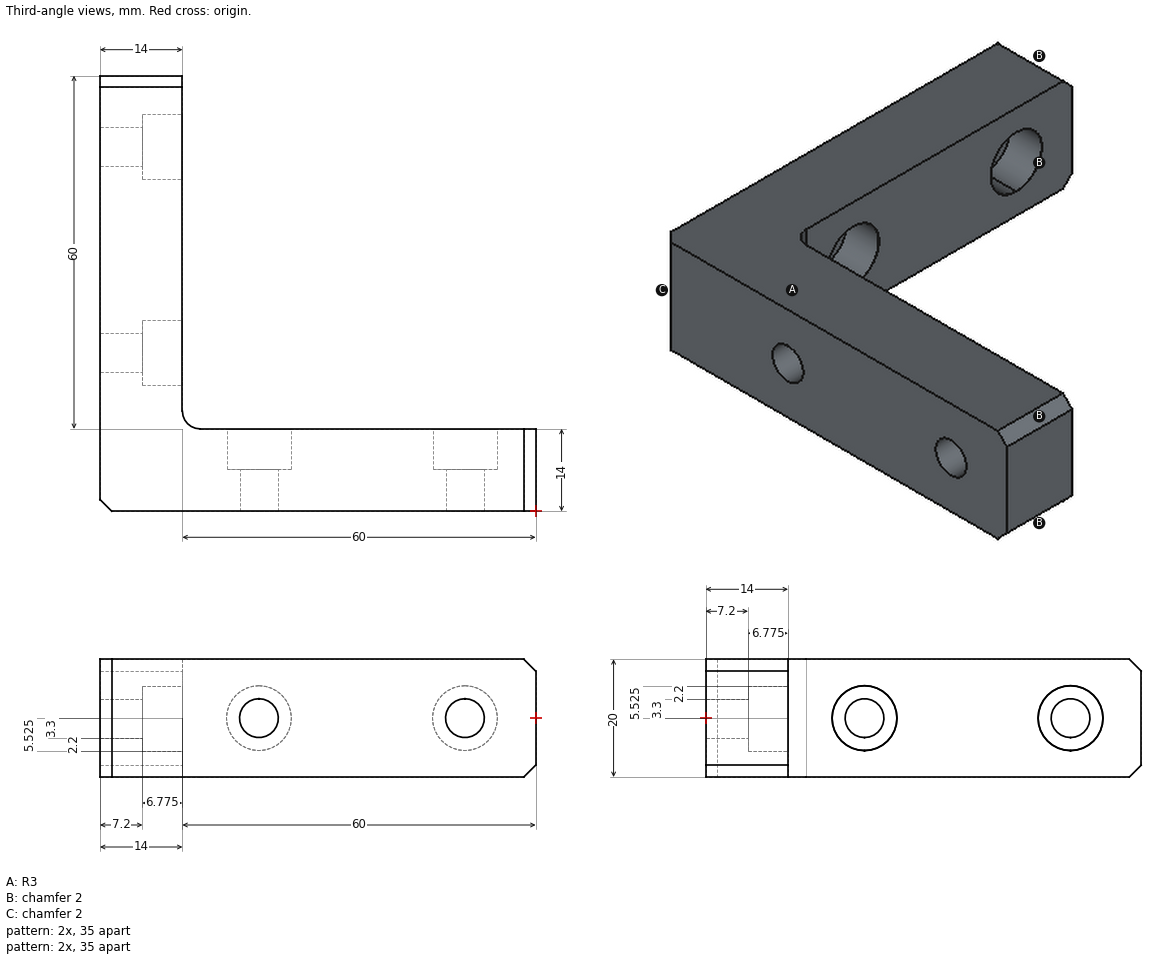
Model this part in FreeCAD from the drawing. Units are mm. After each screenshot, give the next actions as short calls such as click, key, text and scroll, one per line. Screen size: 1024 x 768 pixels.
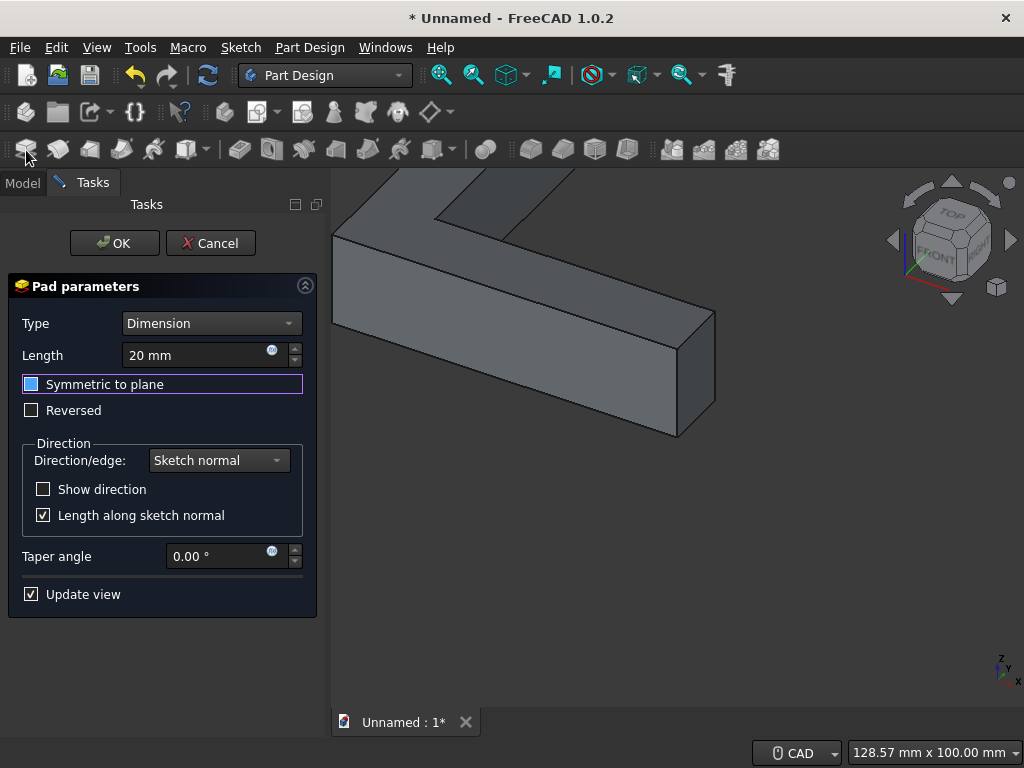
click(30, 384)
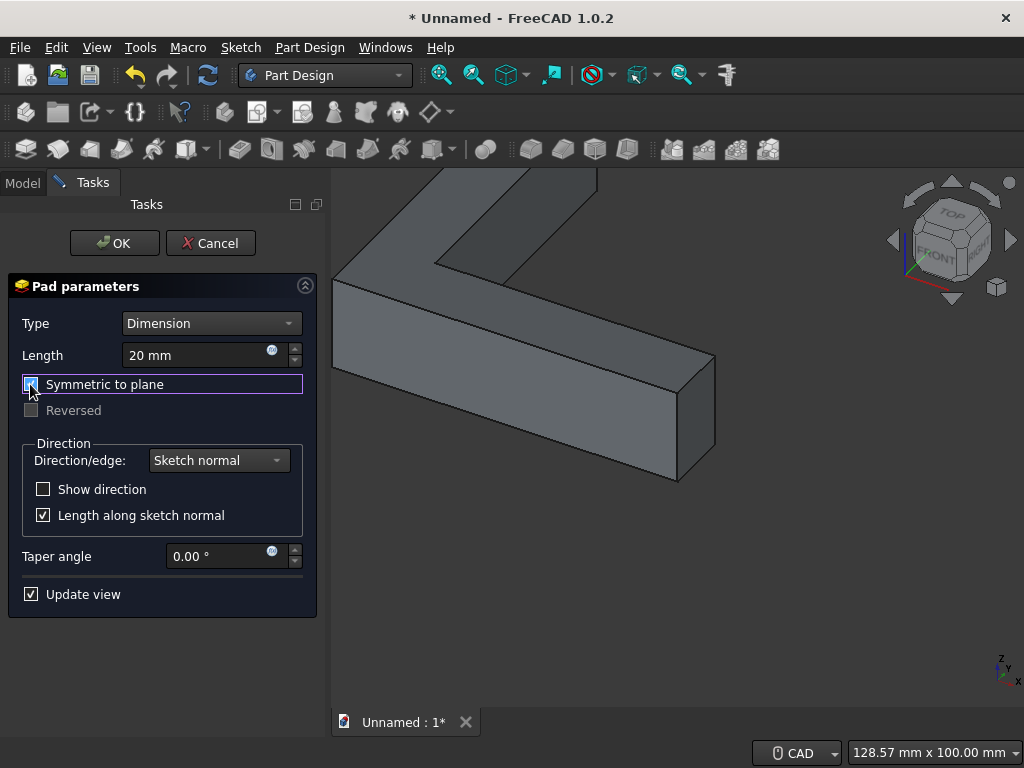
click(115, 243)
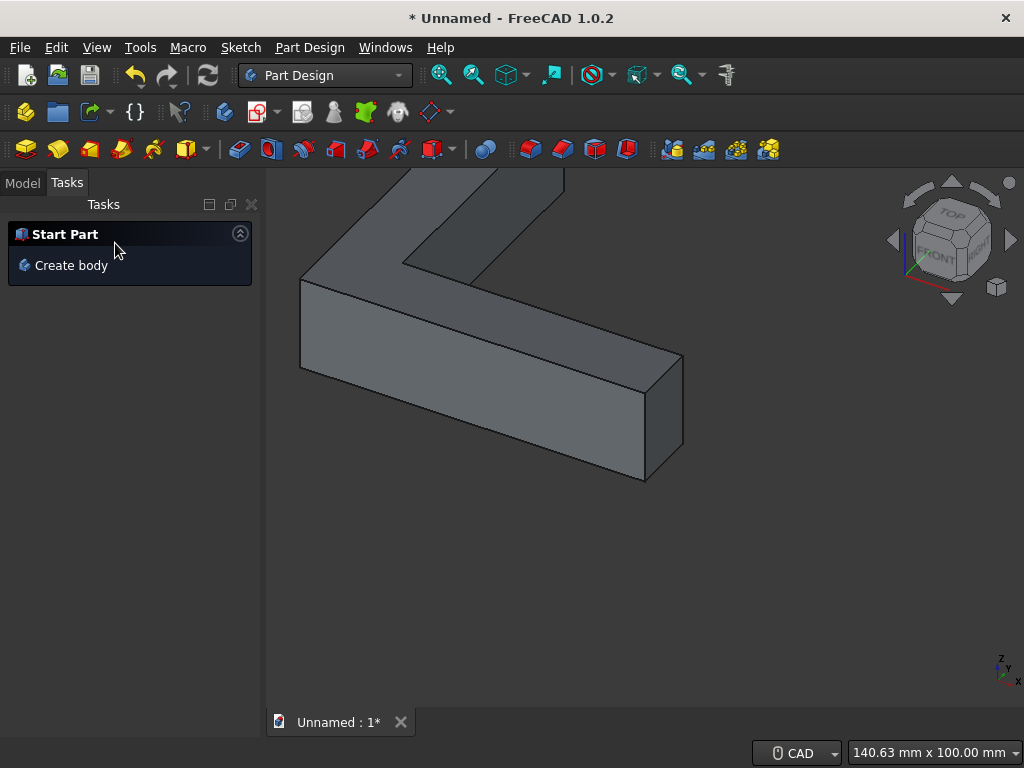
click(442, 76)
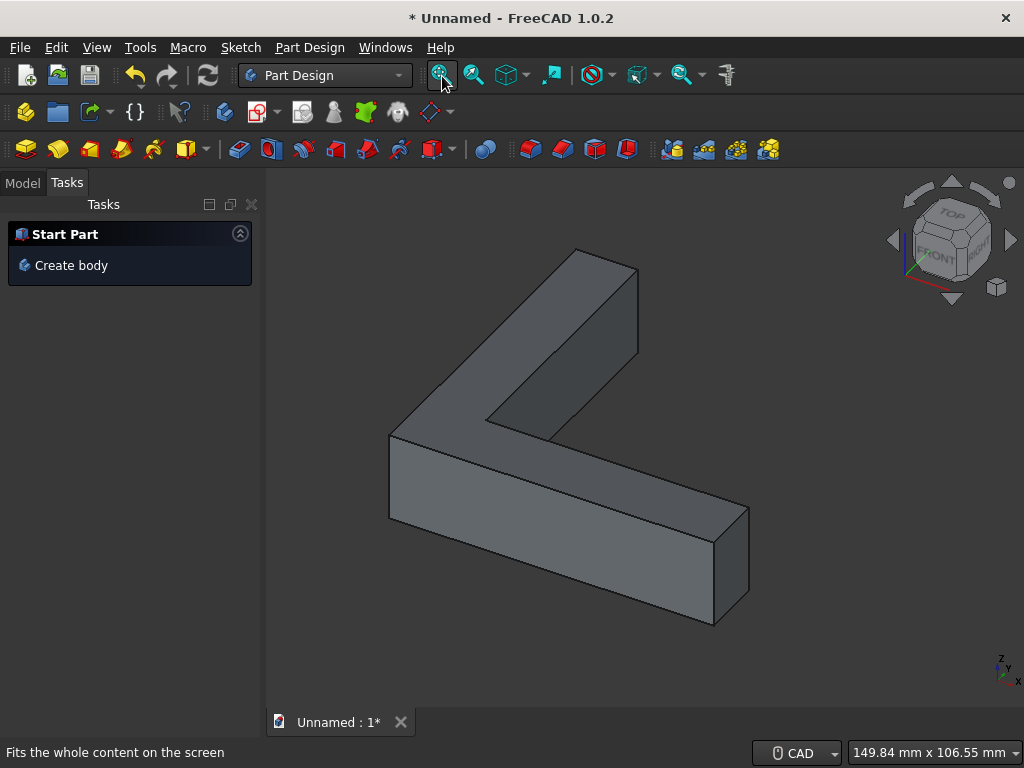
key(0)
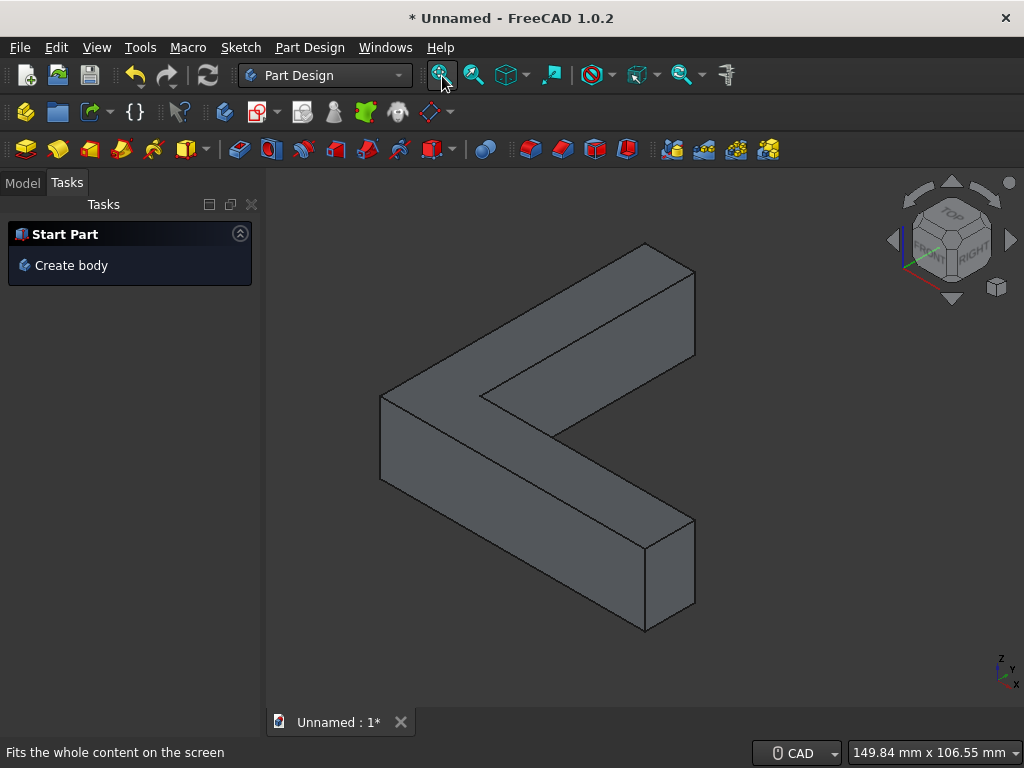
key(2)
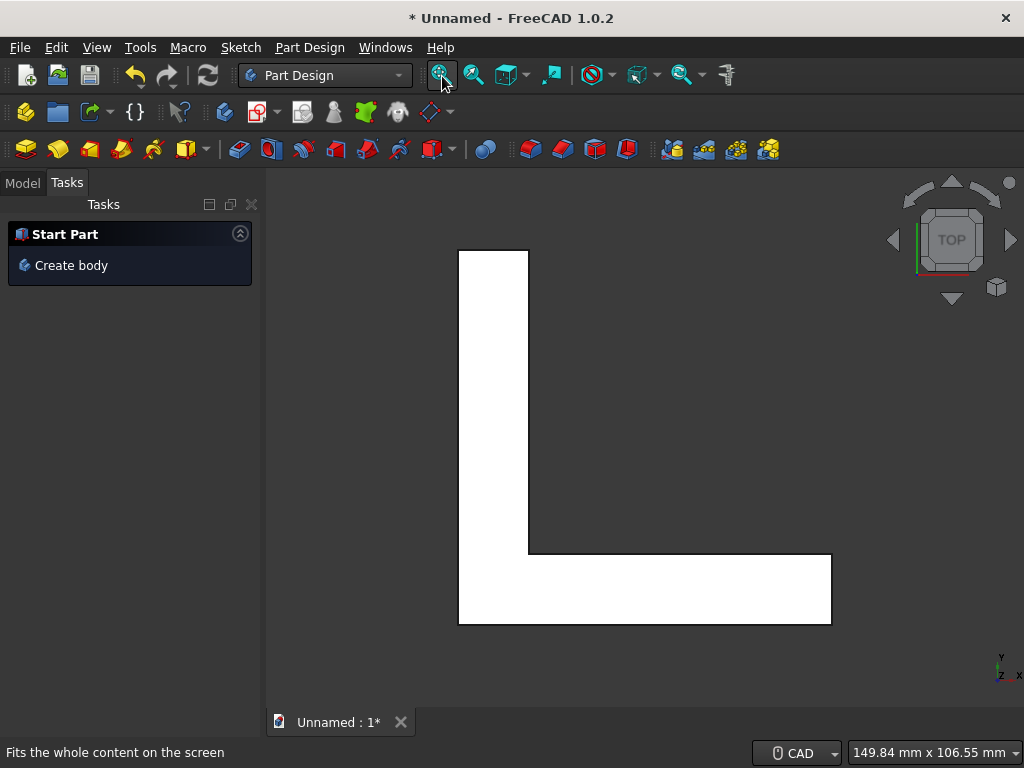
key(1)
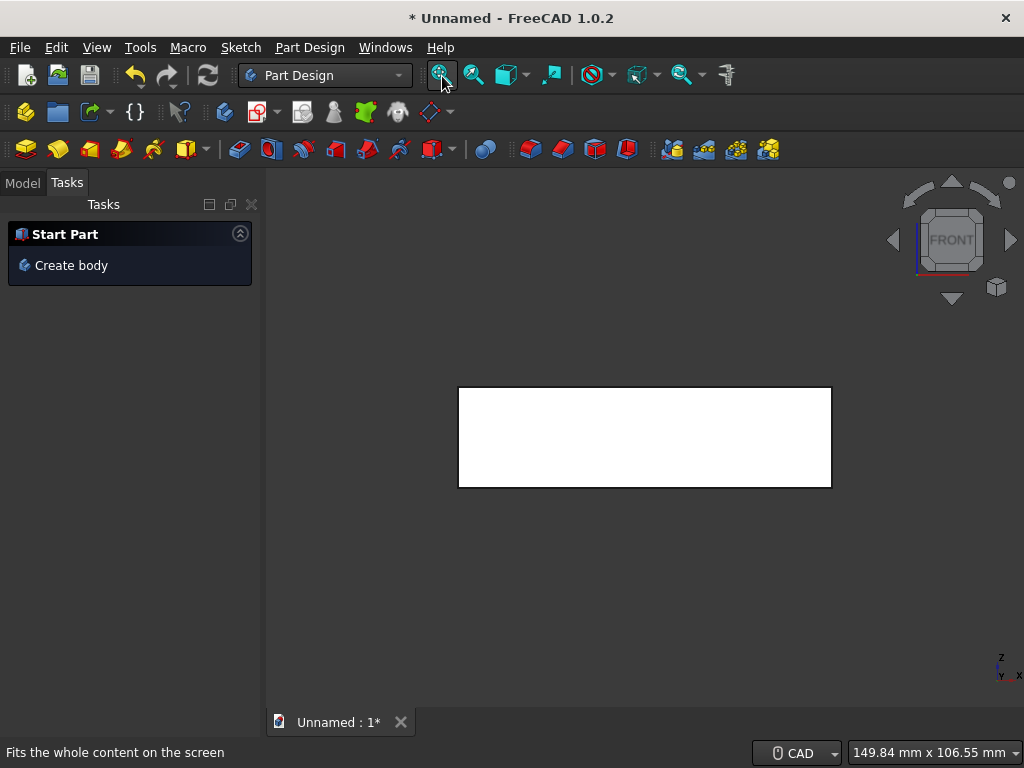
key(3)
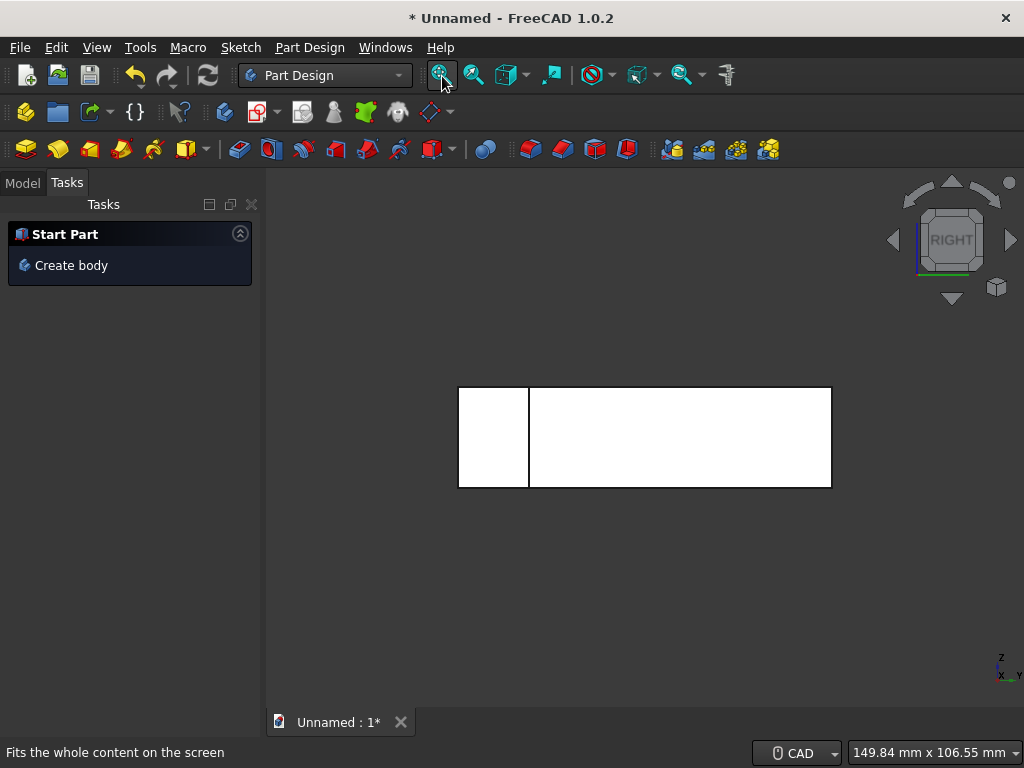
key(5)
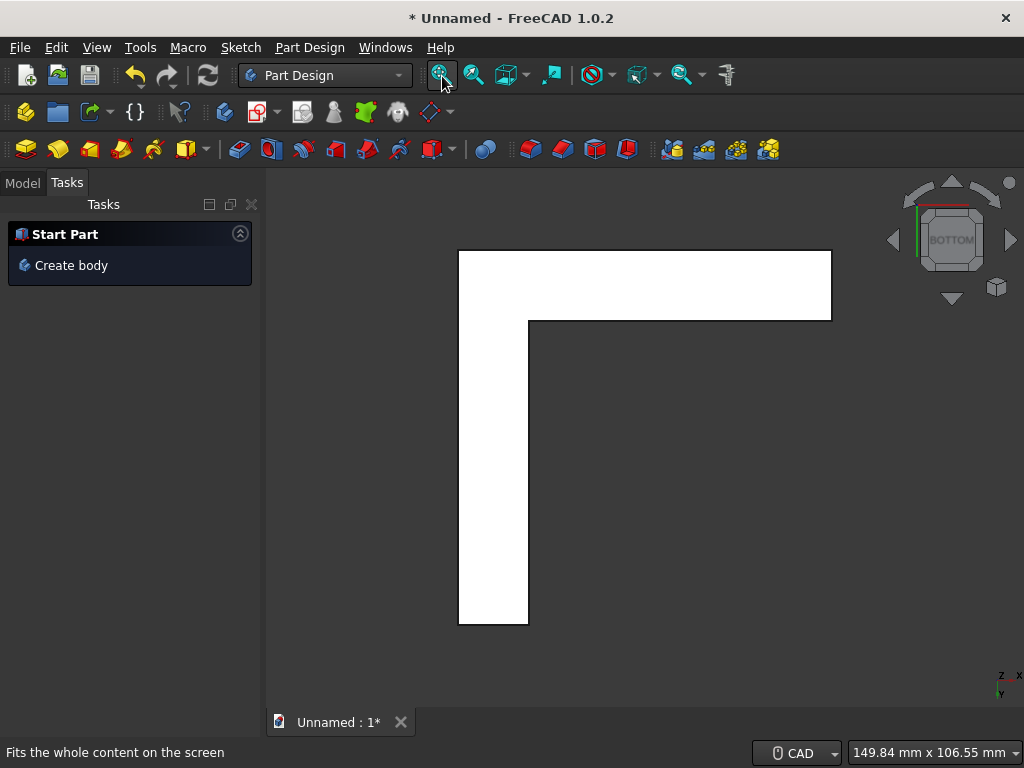
key(4)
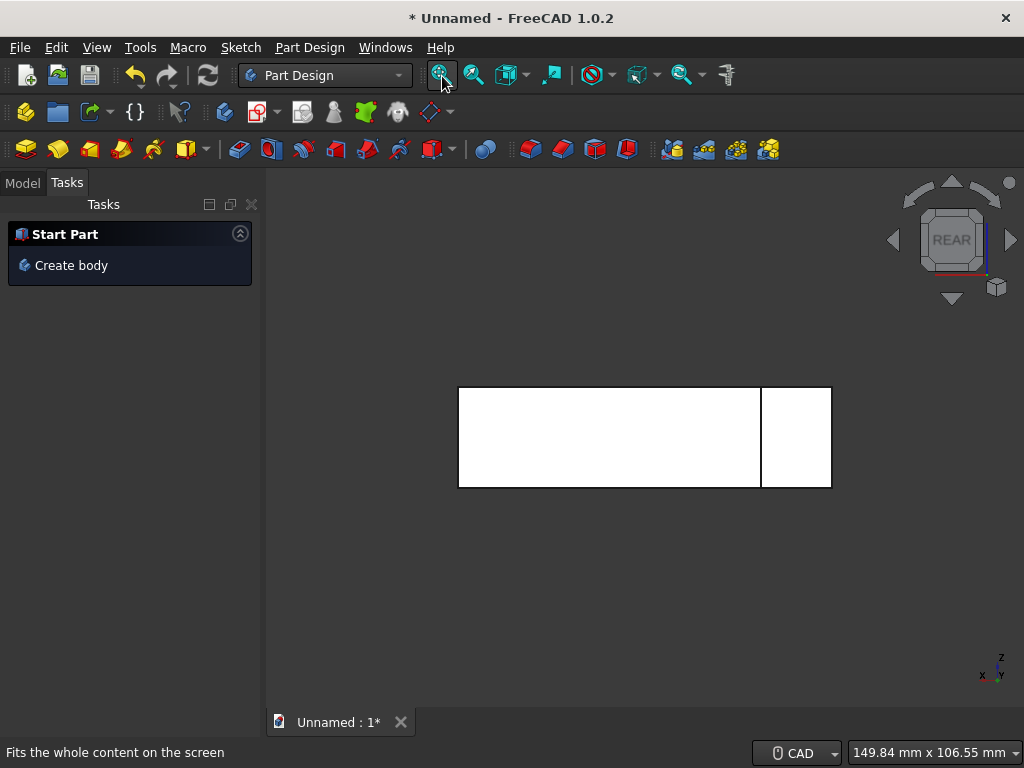
key(6)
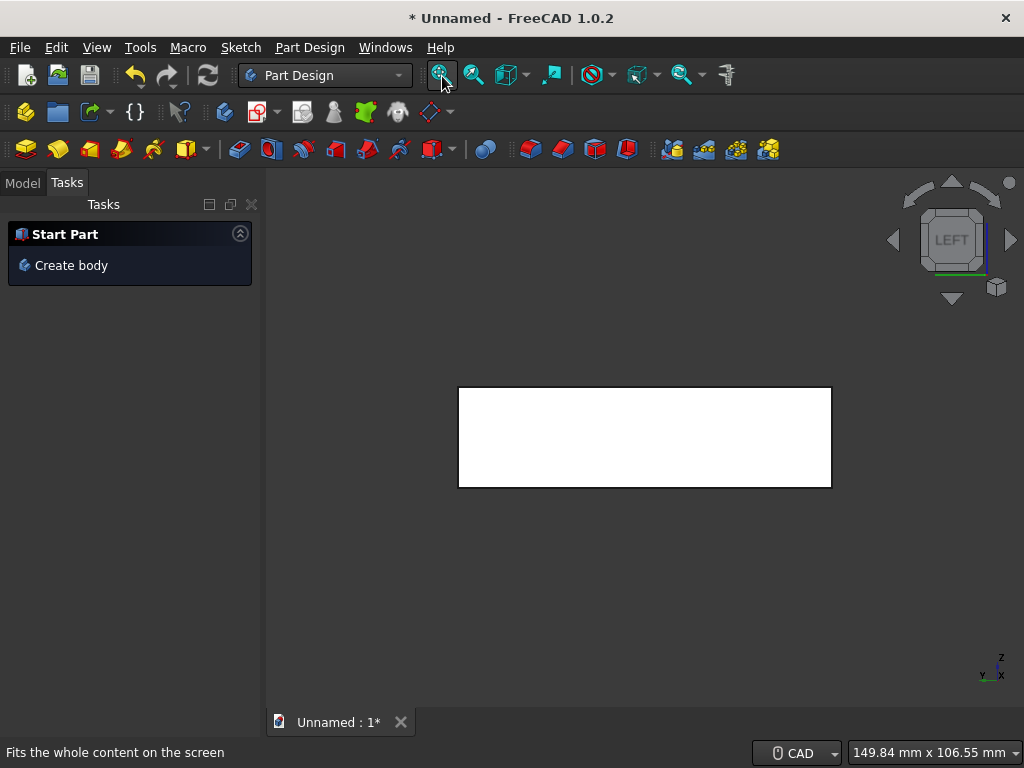
key(v)
key(3)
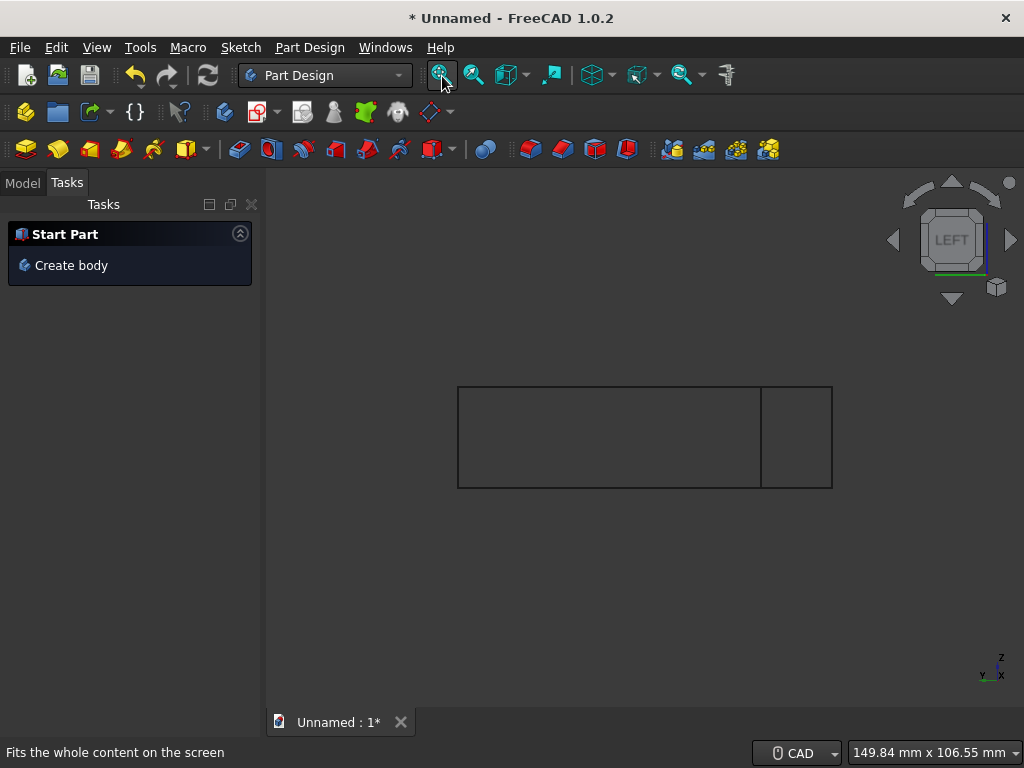
key(0)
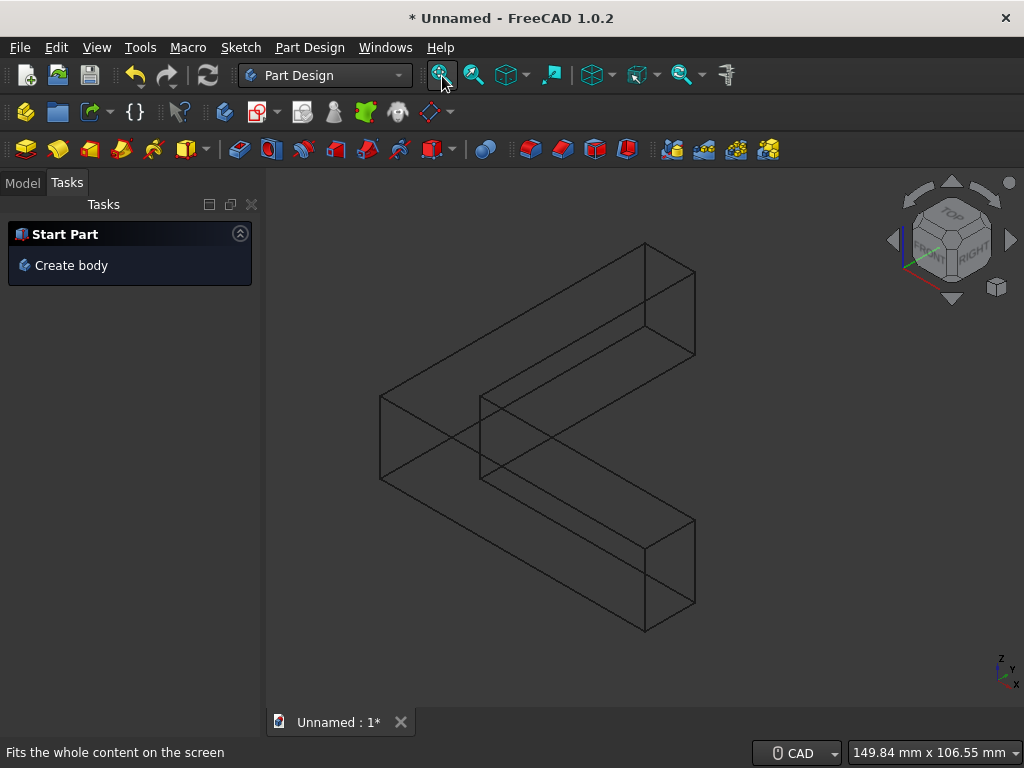
click(480, 436)